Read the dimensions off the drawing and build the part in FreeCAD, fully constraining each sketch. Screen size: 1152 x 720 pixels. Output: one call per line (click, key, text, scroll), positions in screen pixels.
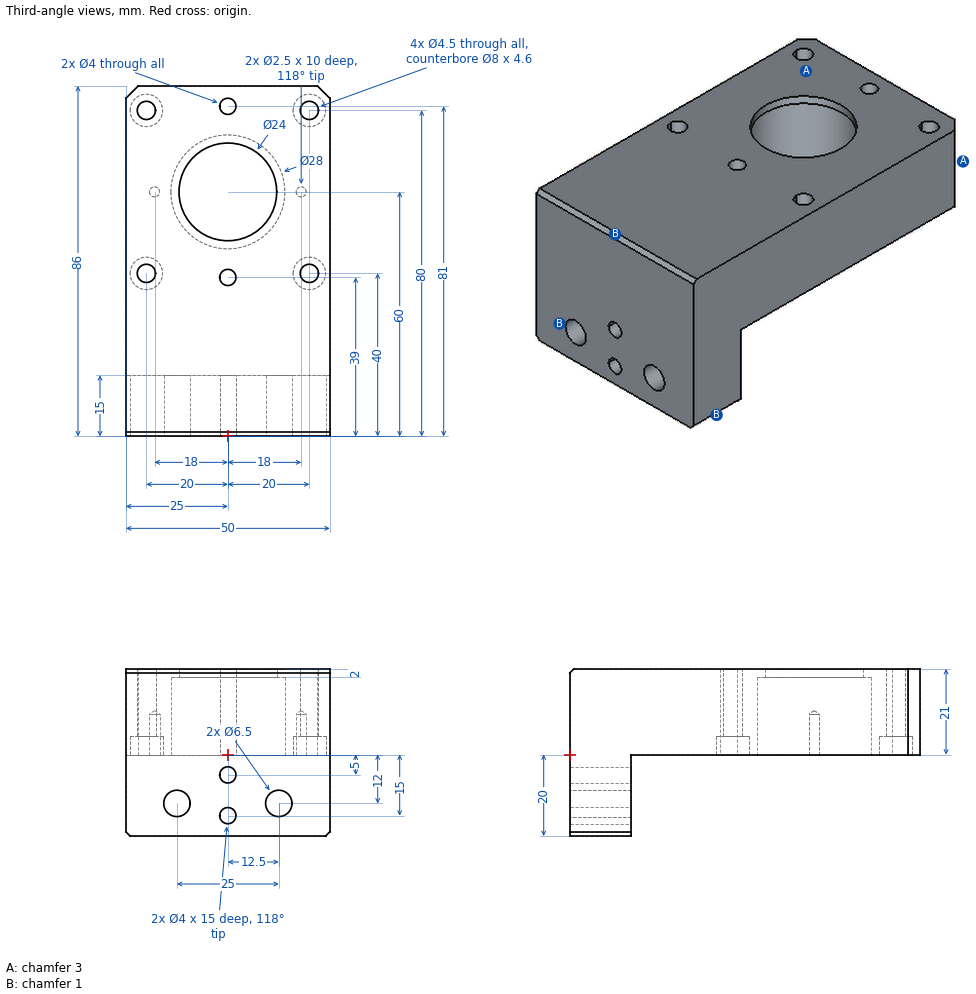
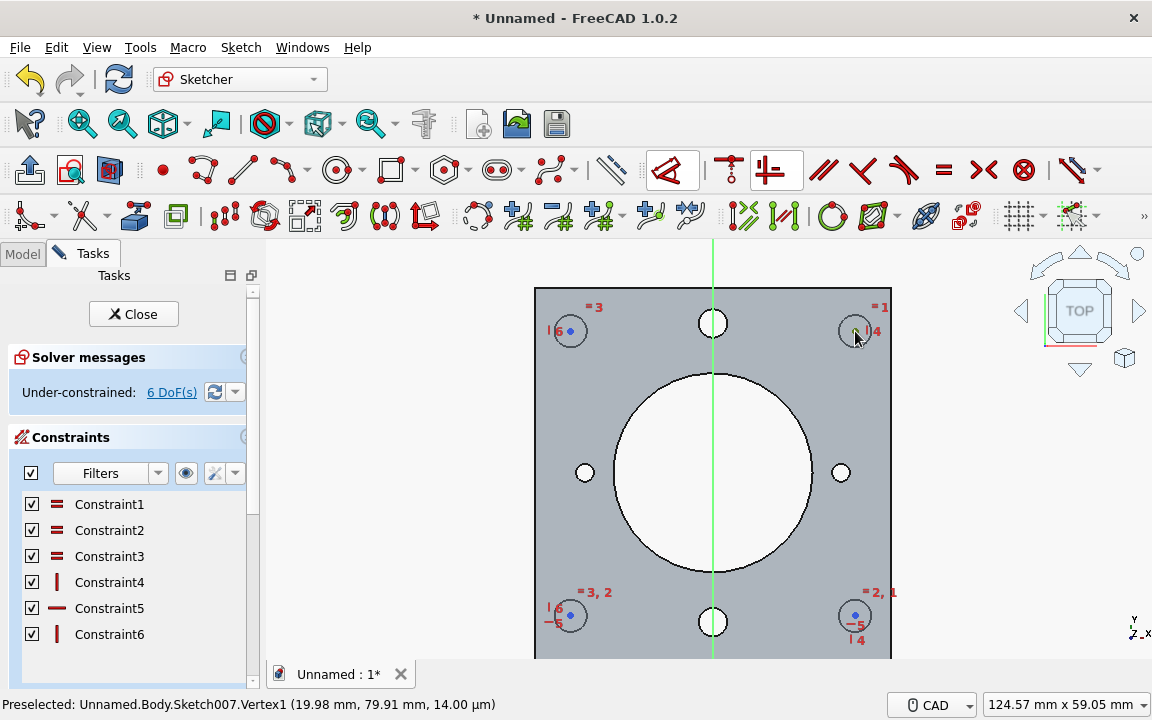
click(571, 331)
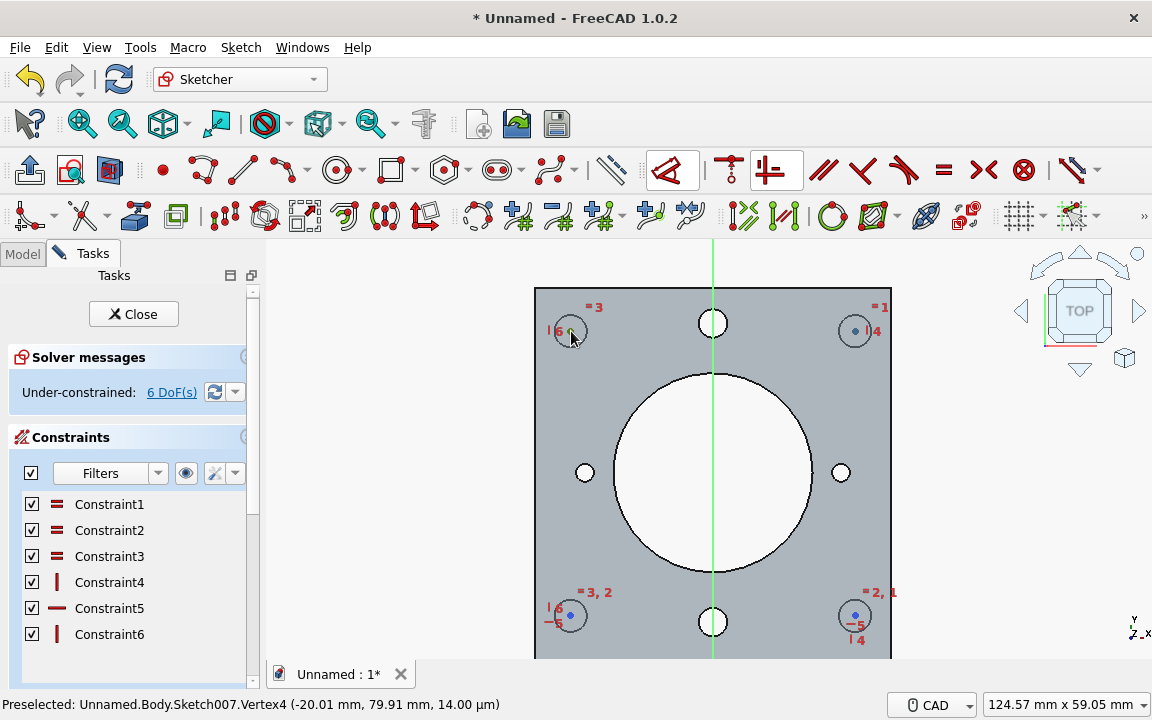
click(798, 170)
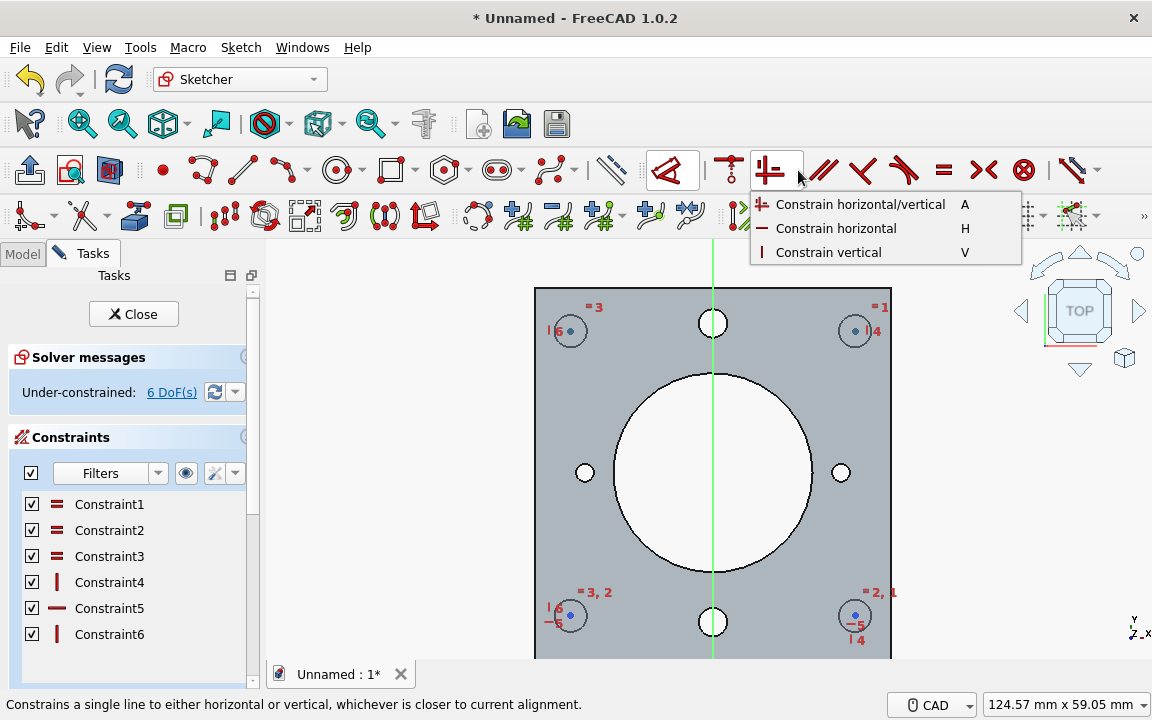
click(886, 228)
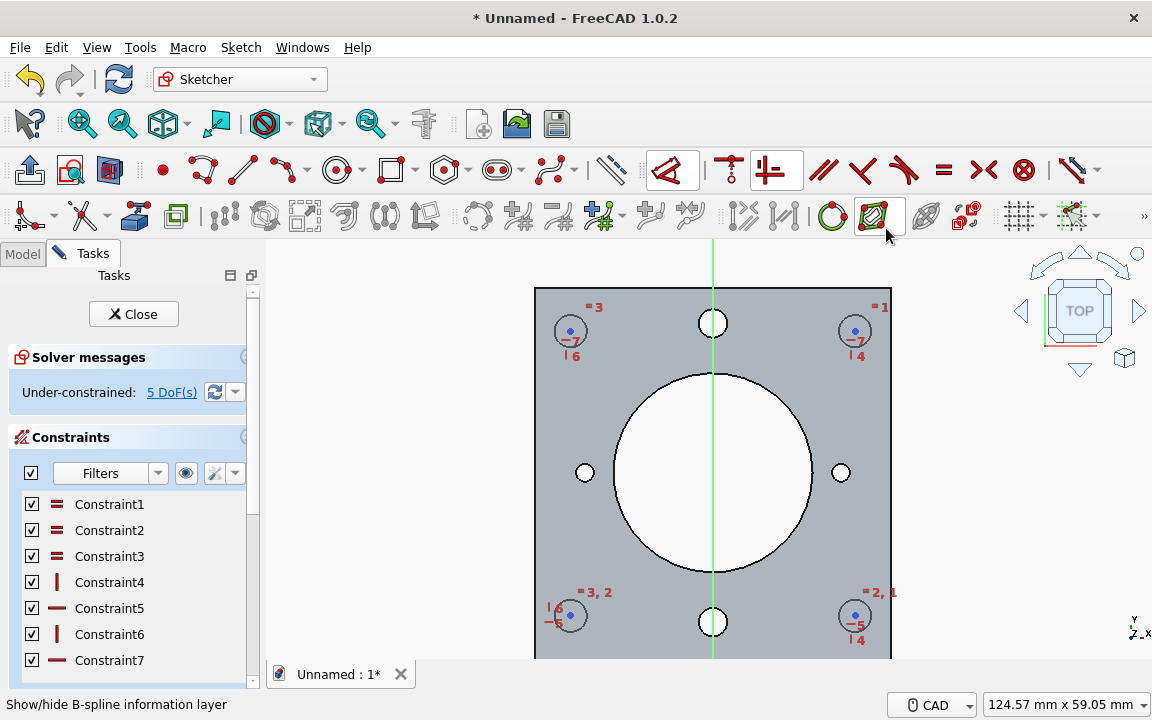
scroll(866, 320, up, 2)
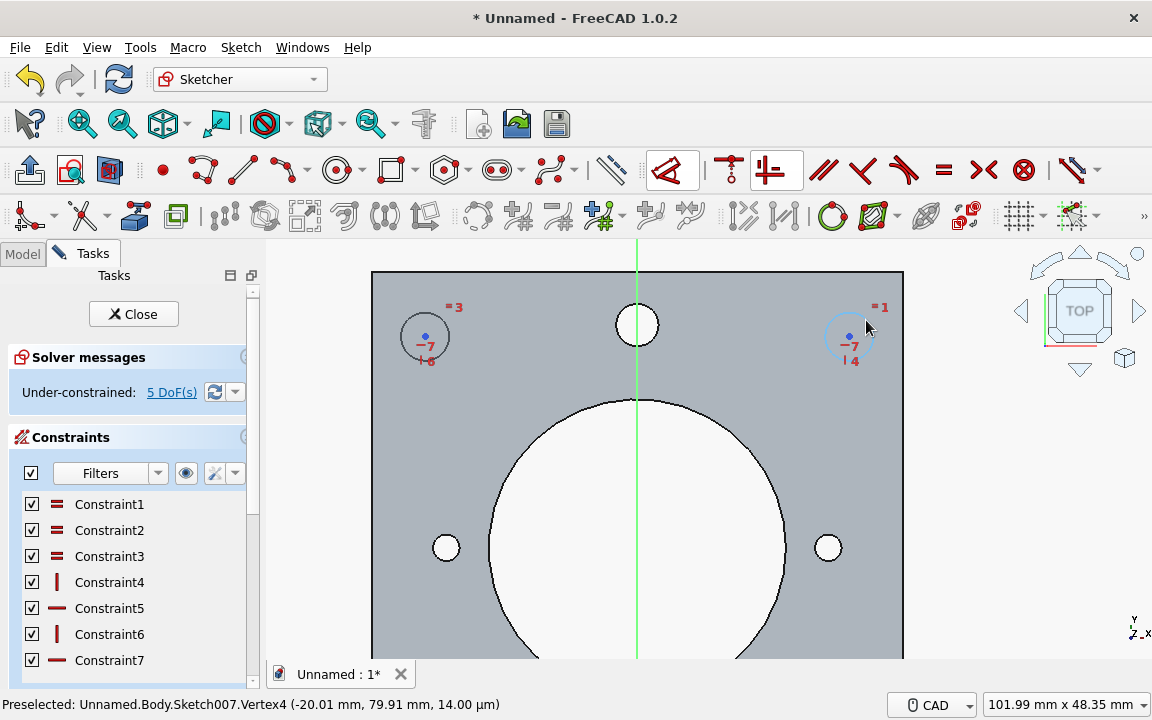
click(866, 320)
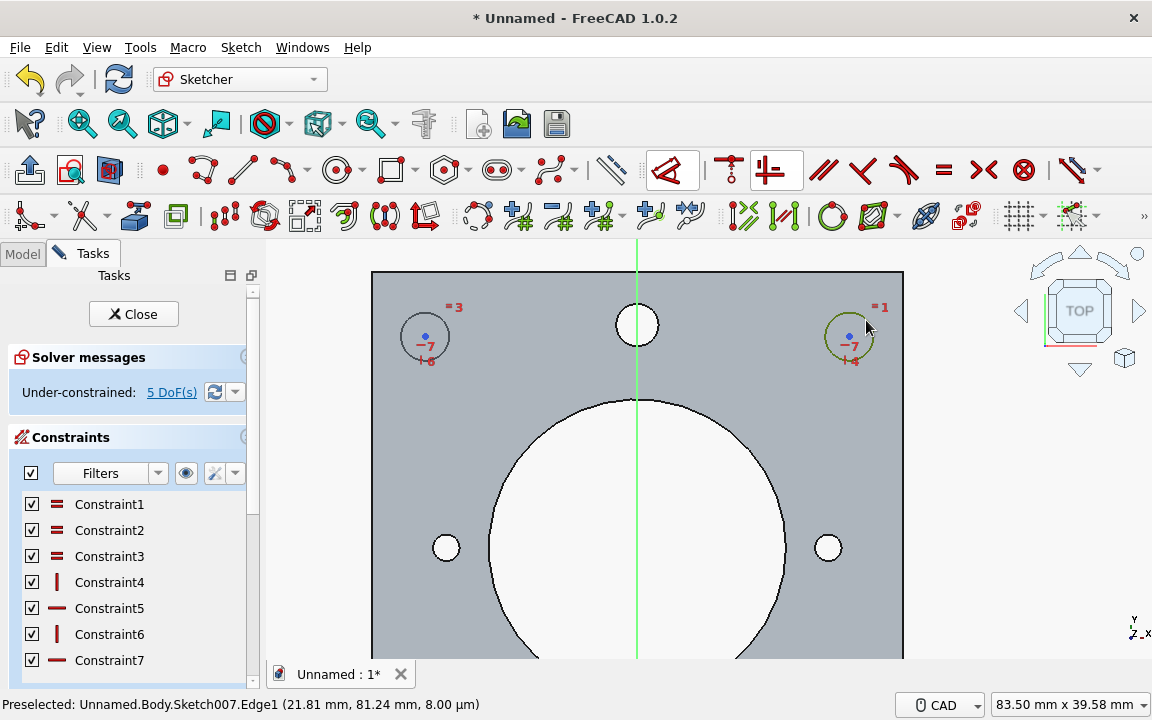
key(k)
key(o)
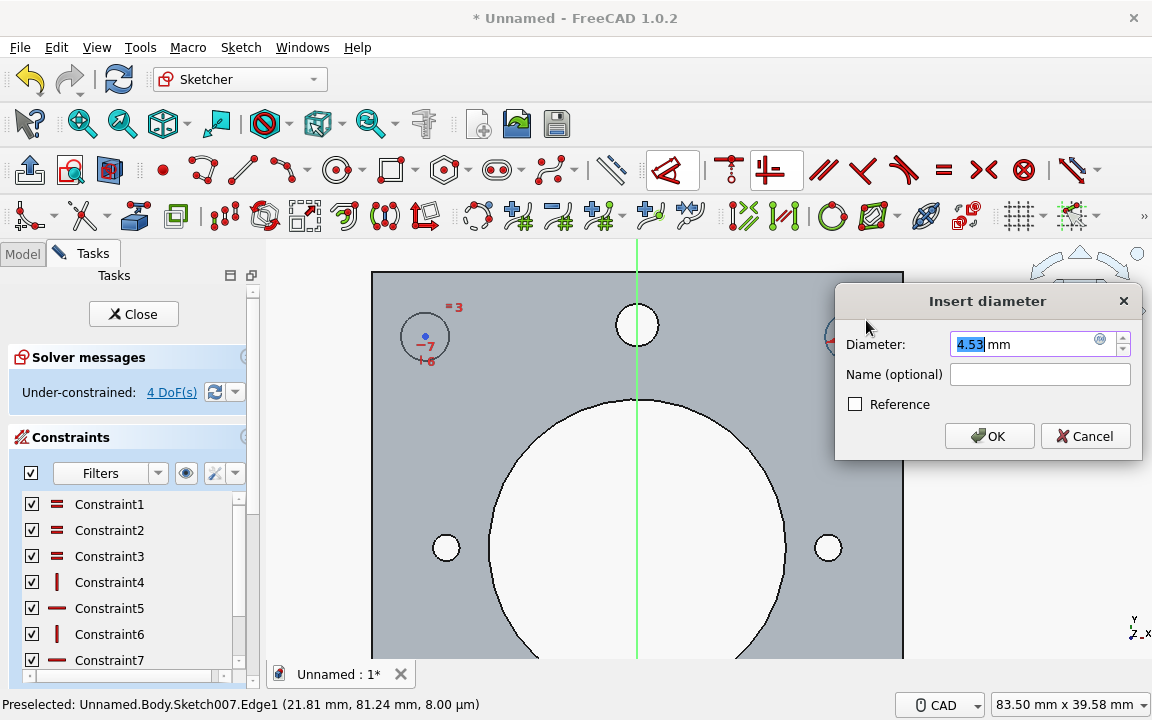
text(4.5)
key(Return)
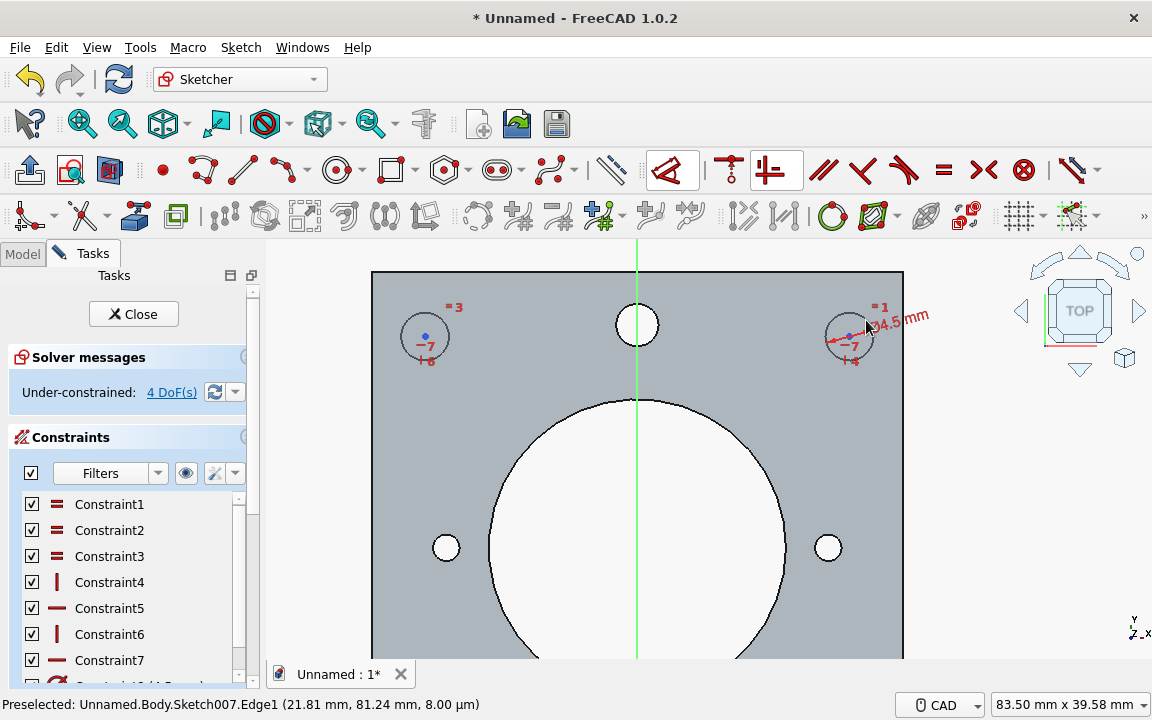
click(849, 337)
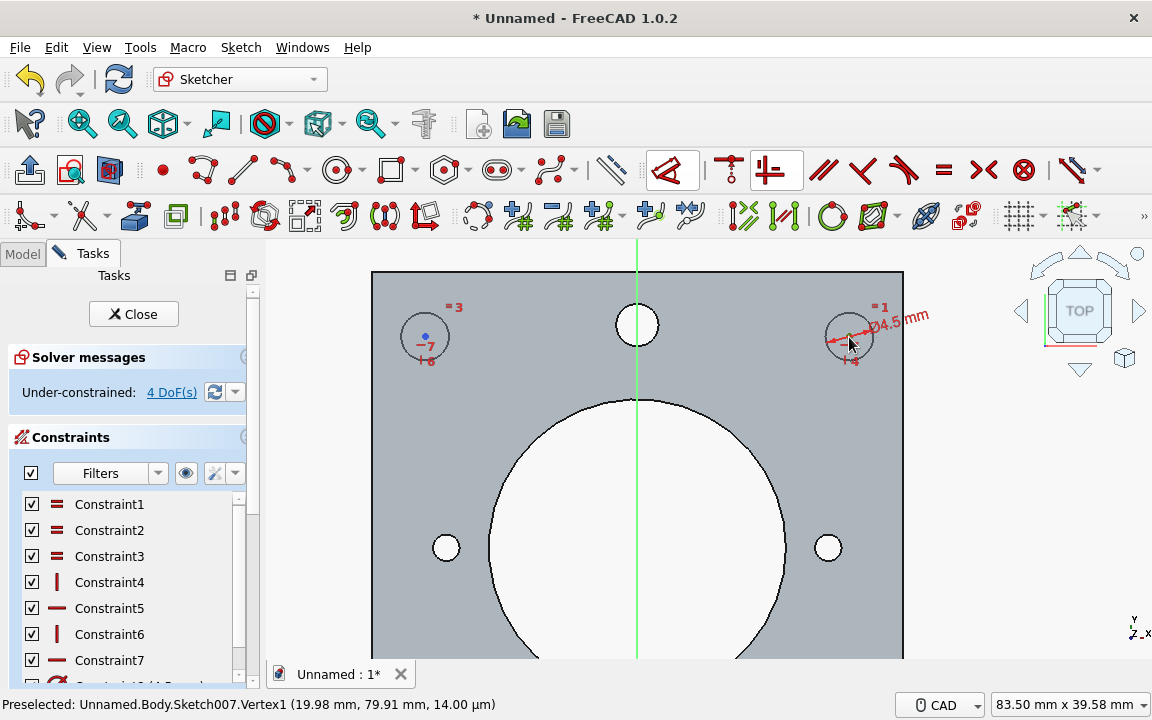
key(l)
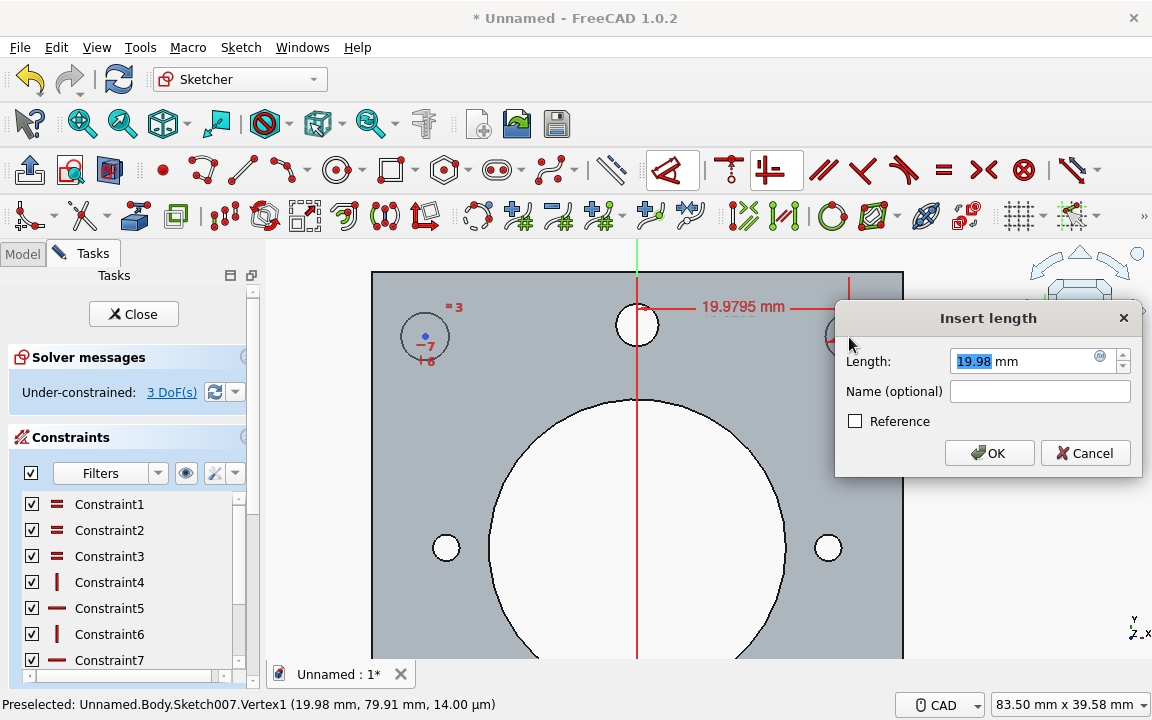
text(20)
key(Return)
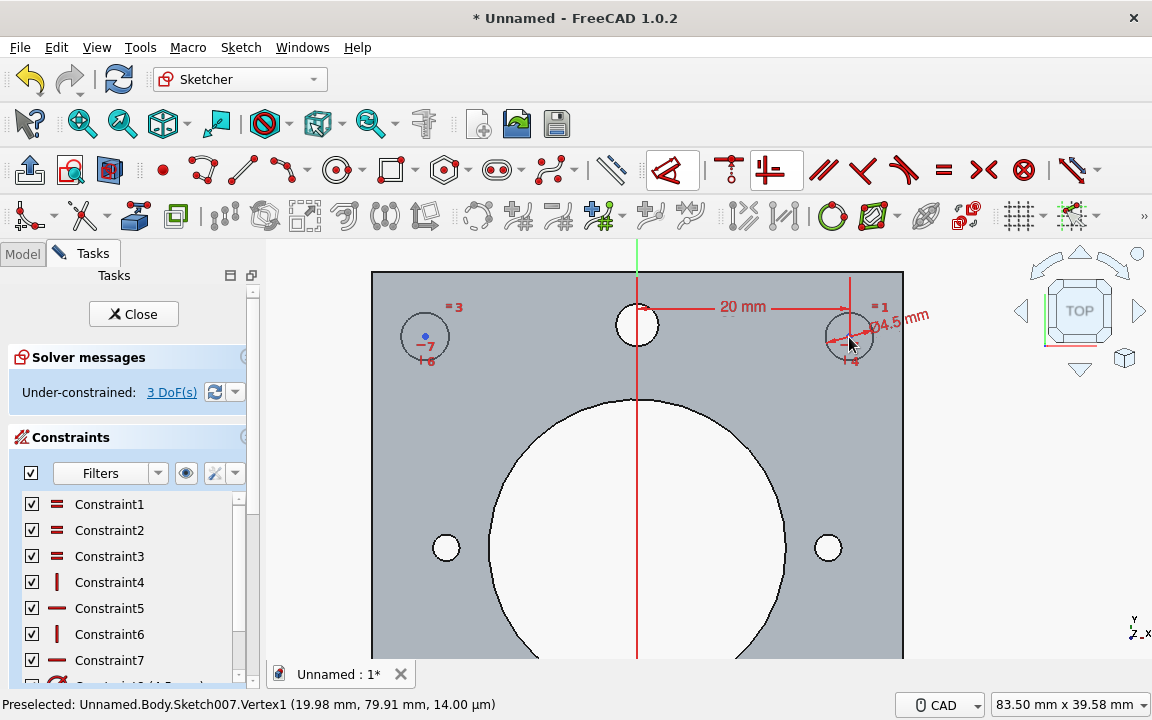
click(850, 337)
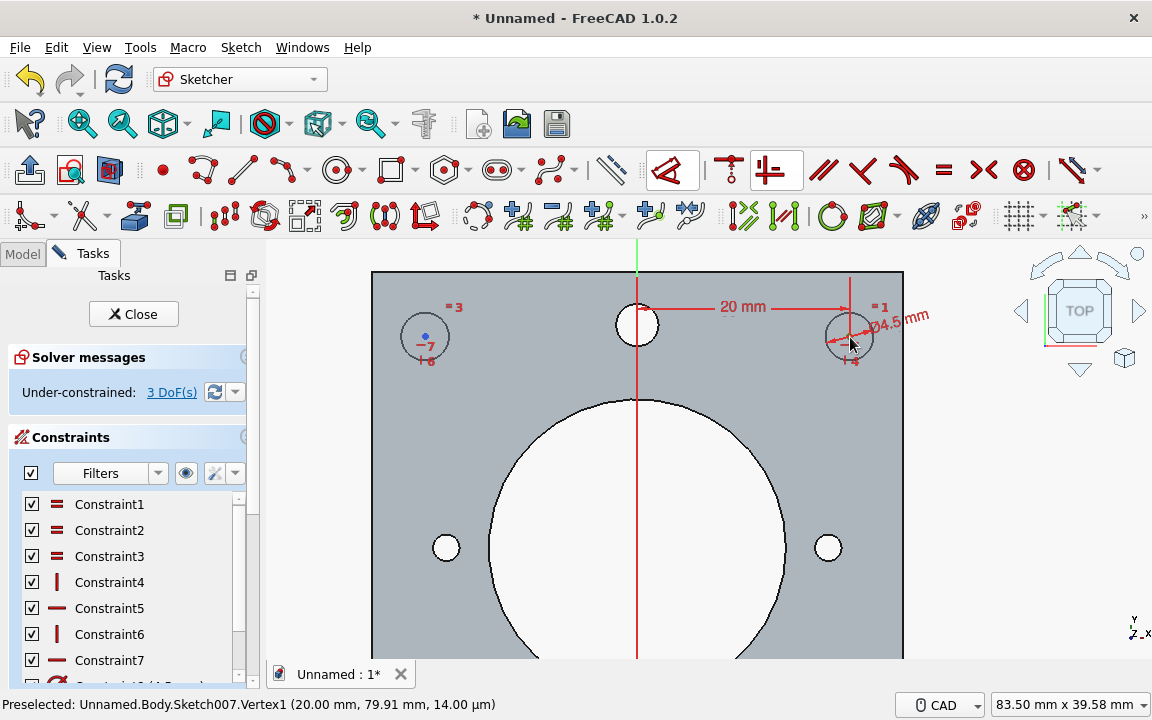
key(i)